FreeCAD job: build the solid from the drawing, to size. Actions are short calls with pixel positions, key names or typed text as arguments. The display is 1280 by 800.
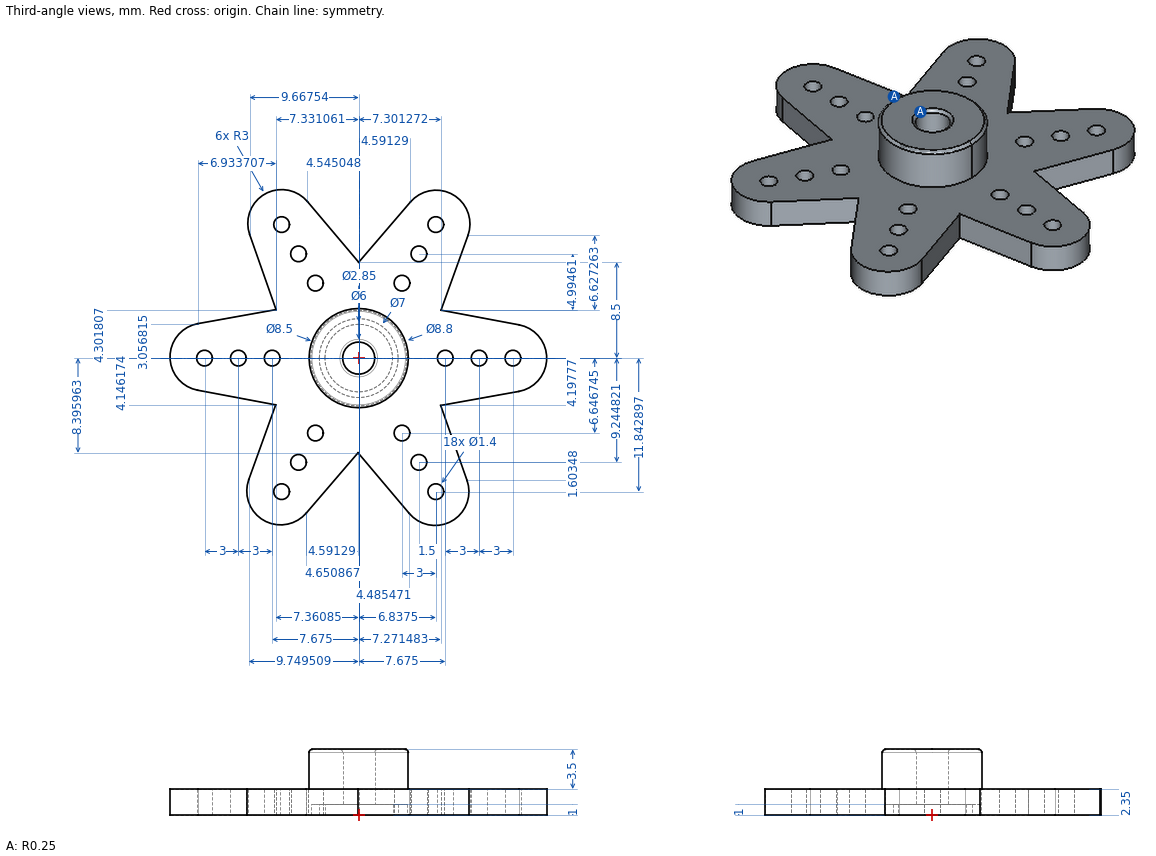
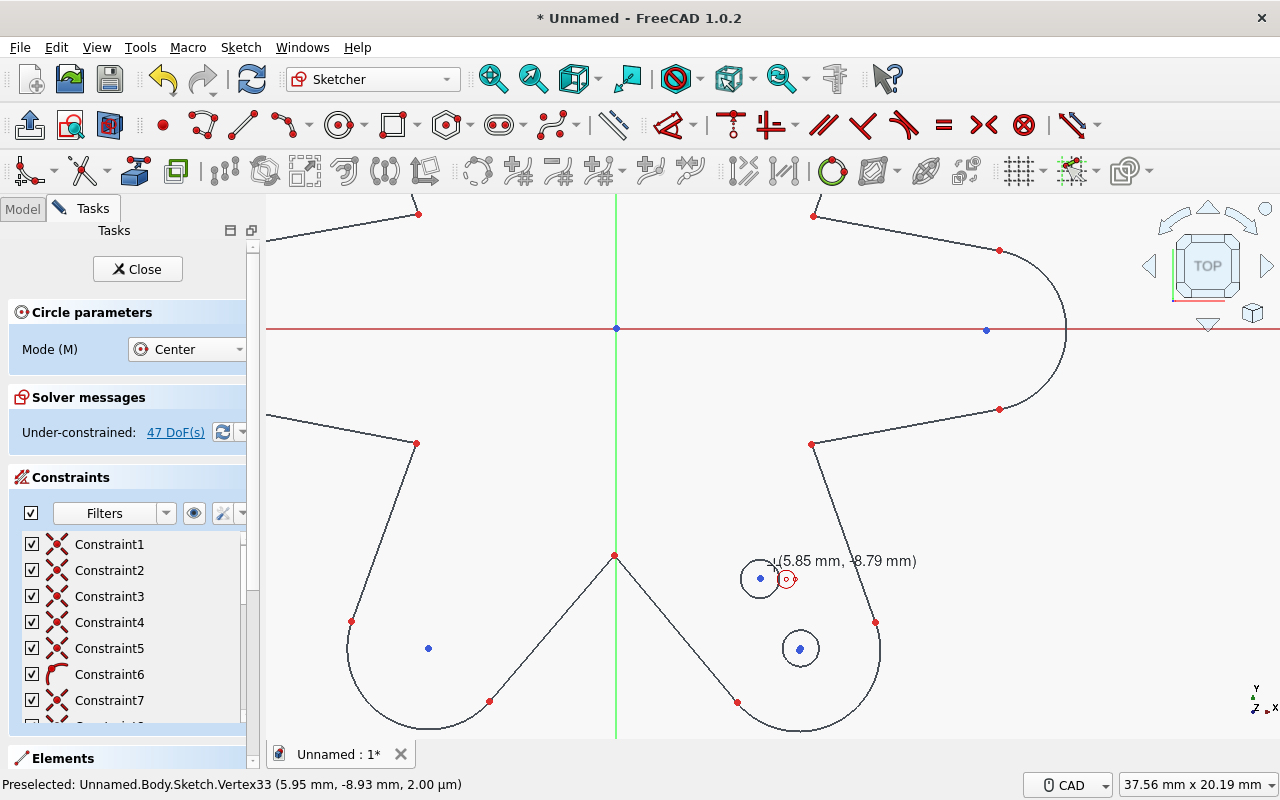
click(720, 508)
click(733, 495)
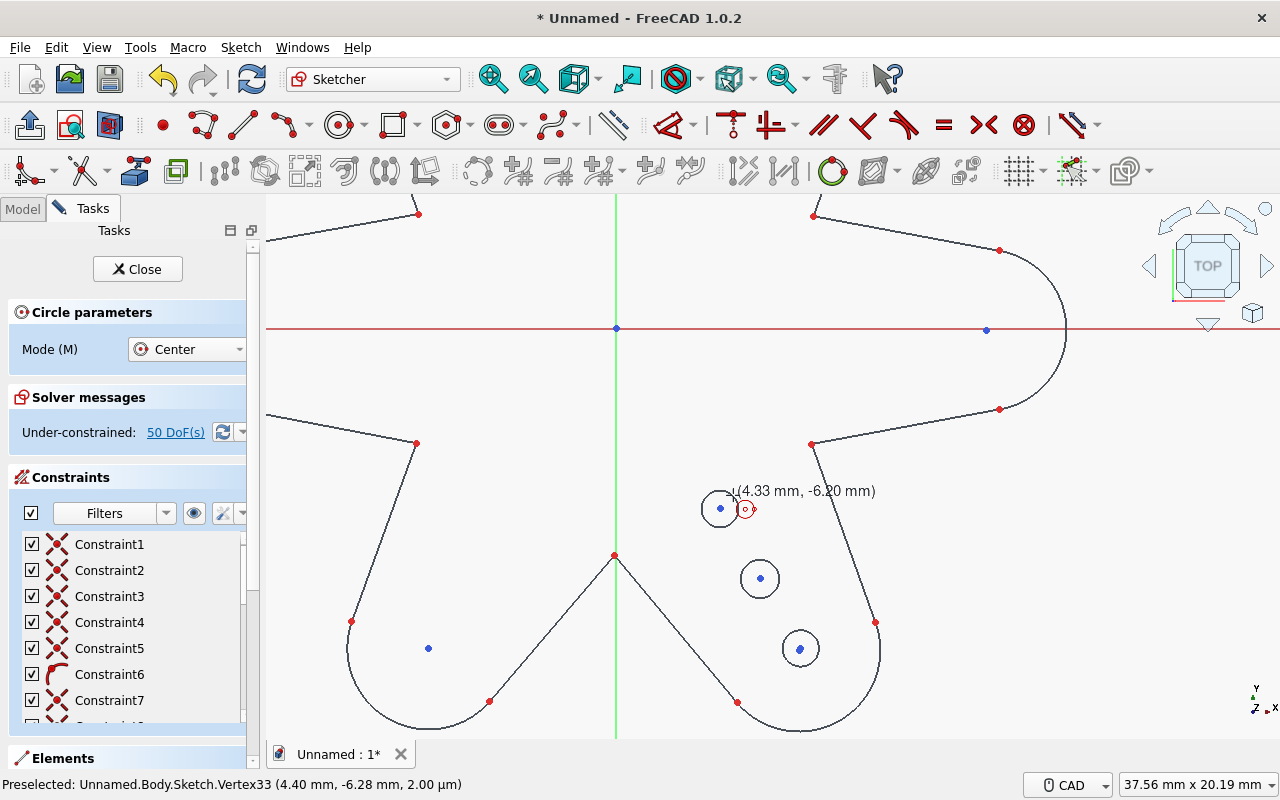
scroll(432, 648, up, 9)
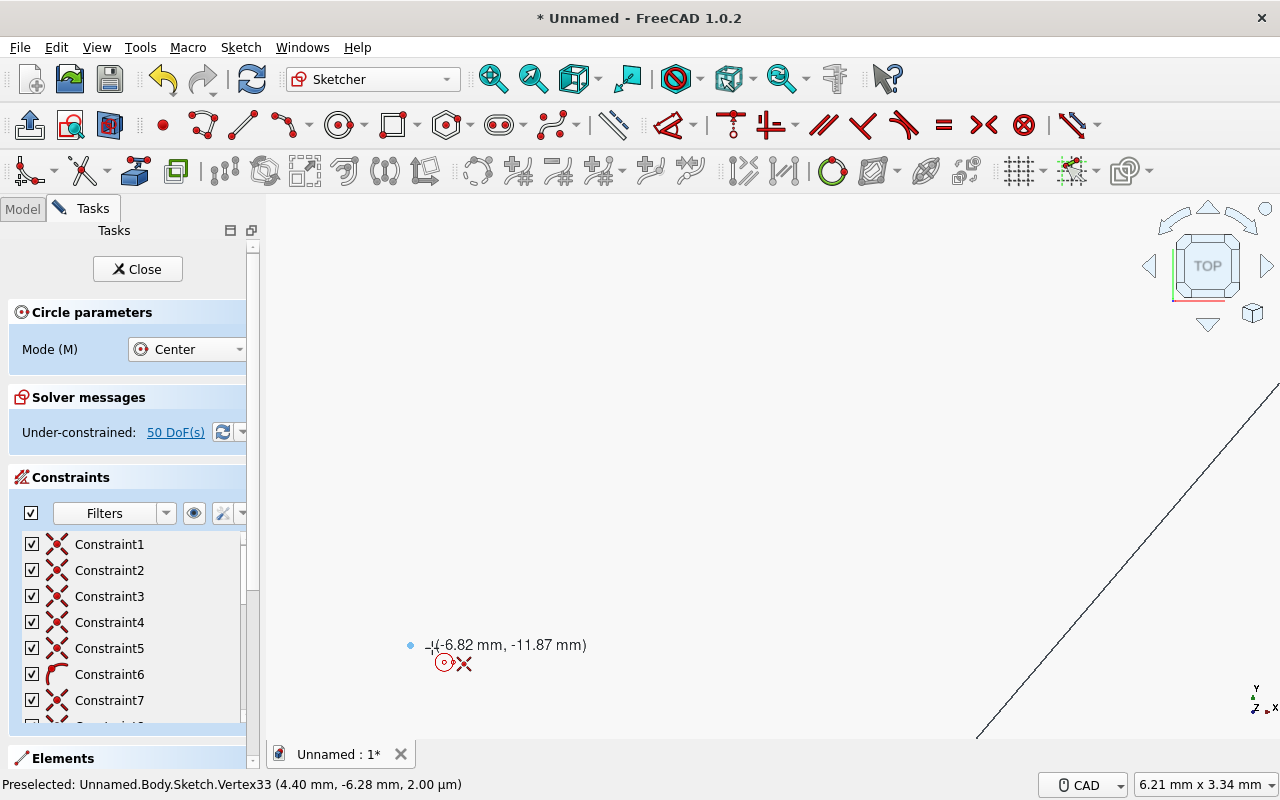
click(428, 646)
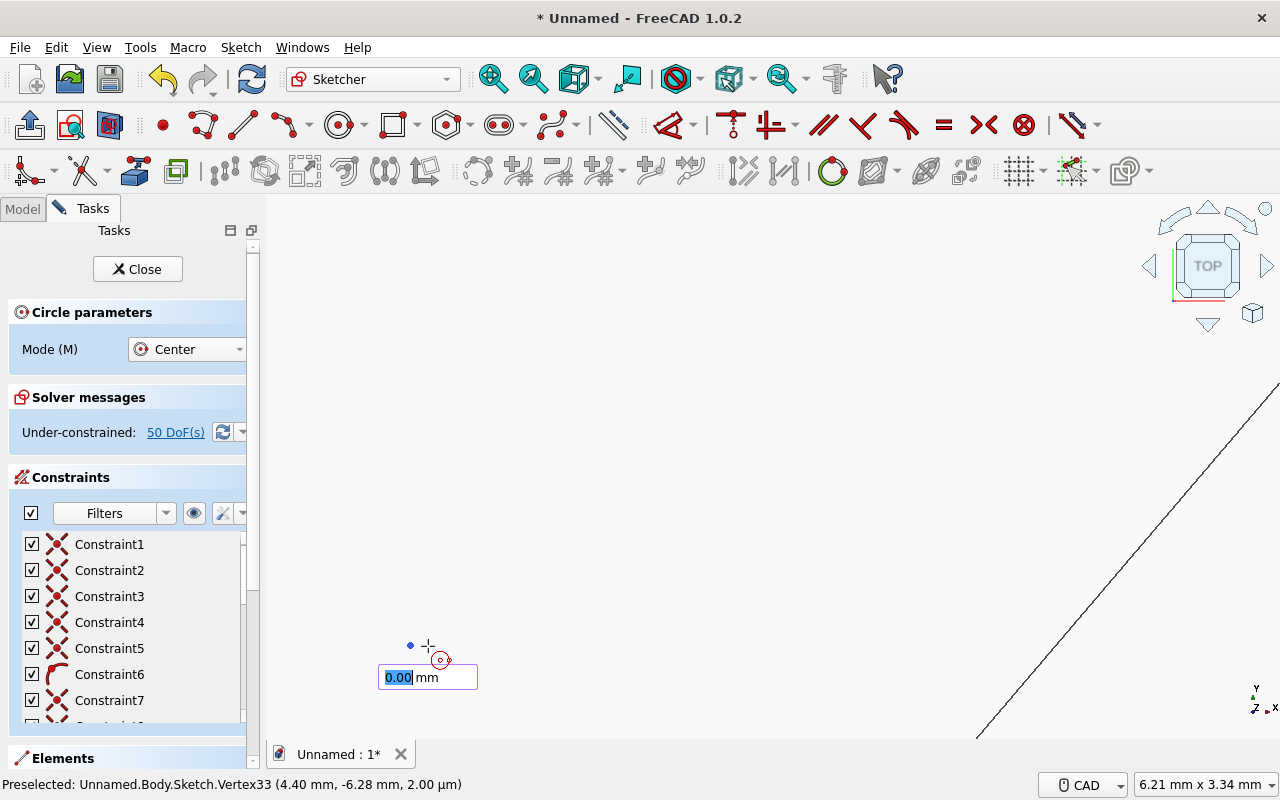
scroll(637, 608, down, 13)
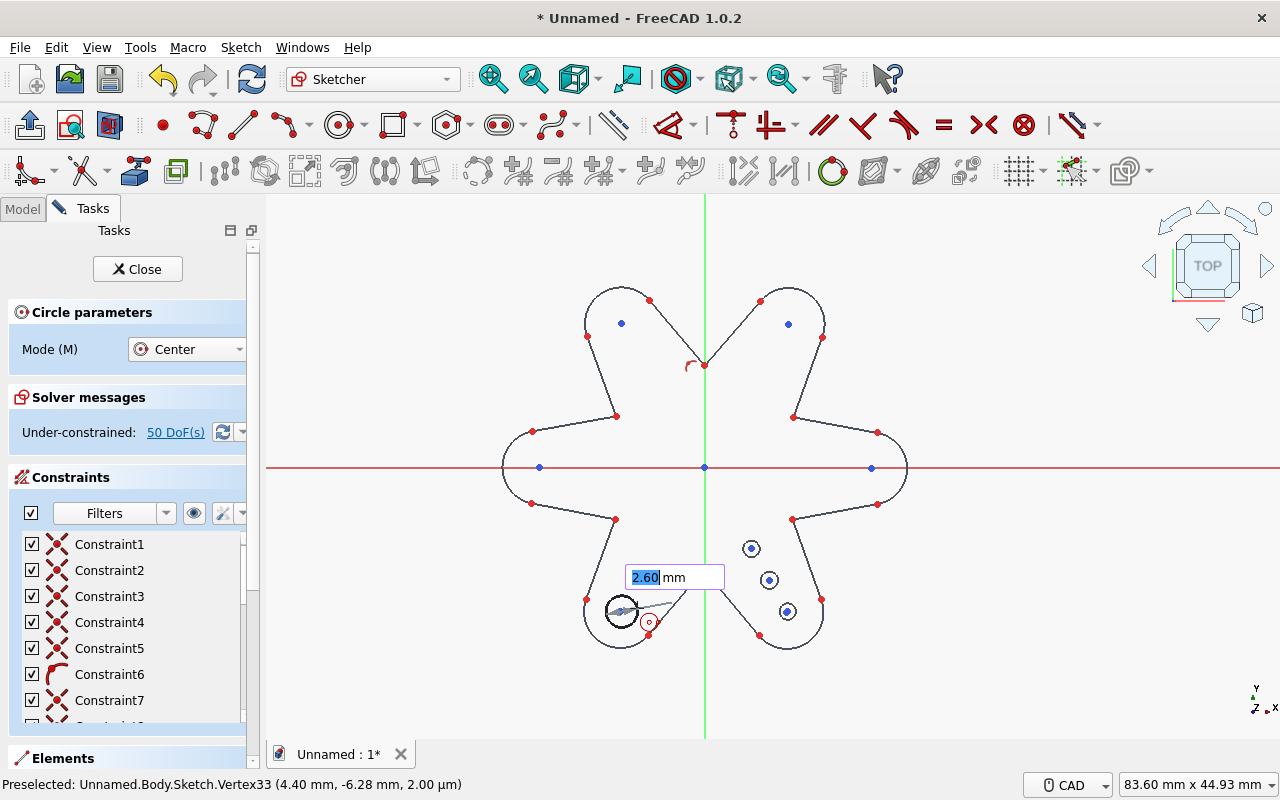
scroll(628, 605, up, 4)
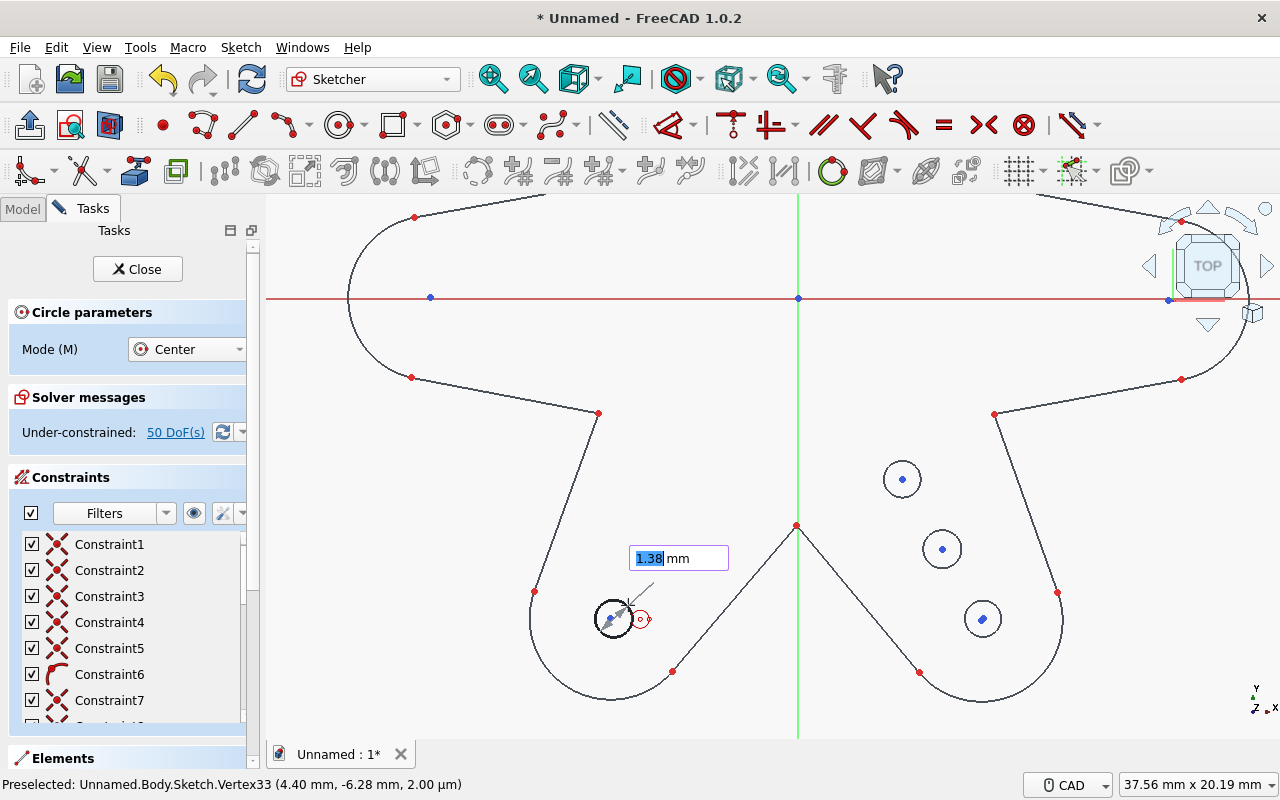
click(627, 605)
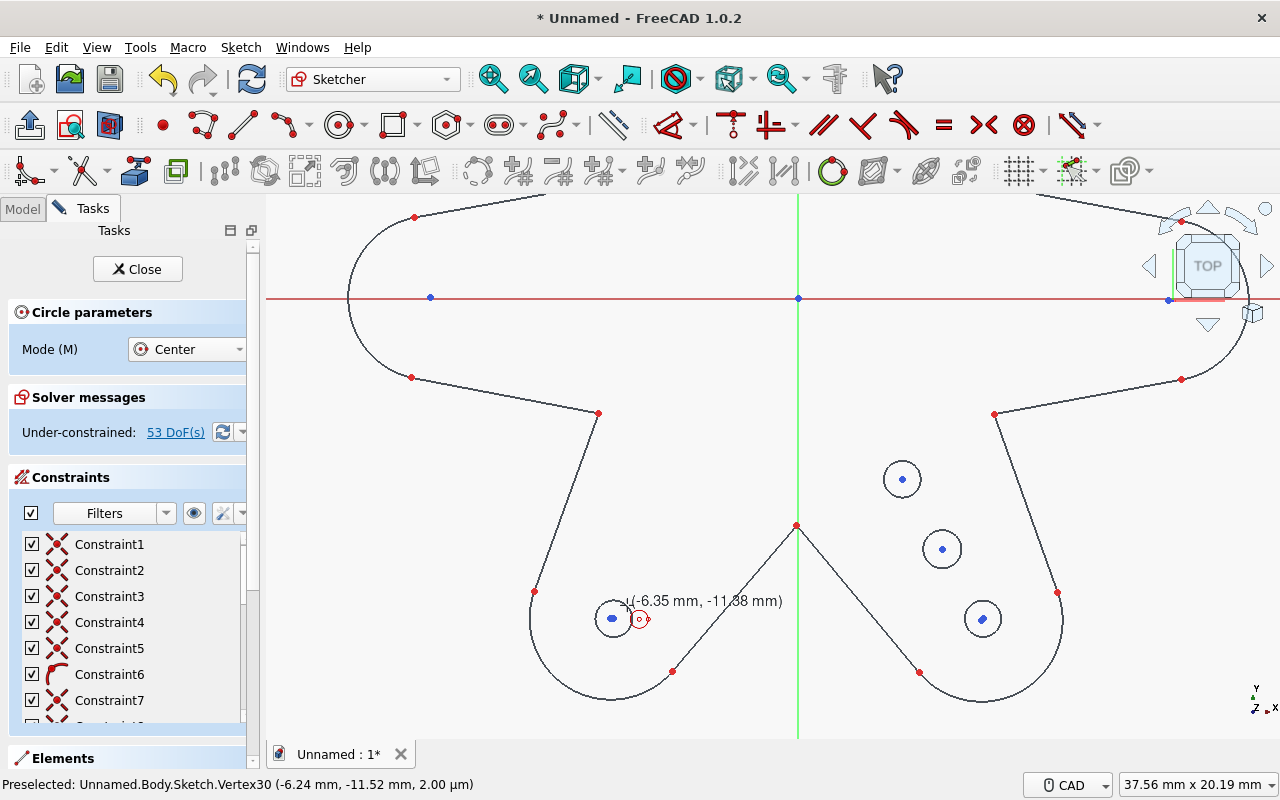
click(654, 548)
click(668, 535)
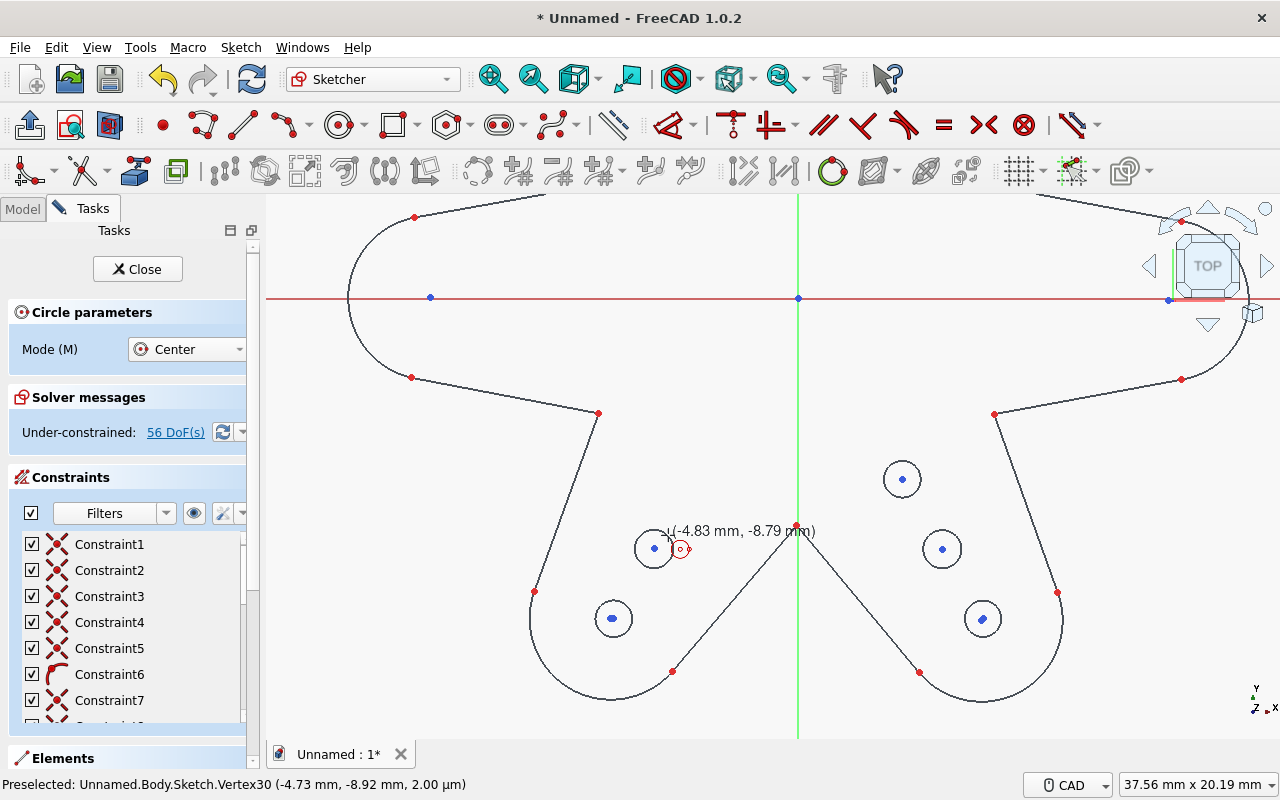
click(695, 478)
click(708, 465)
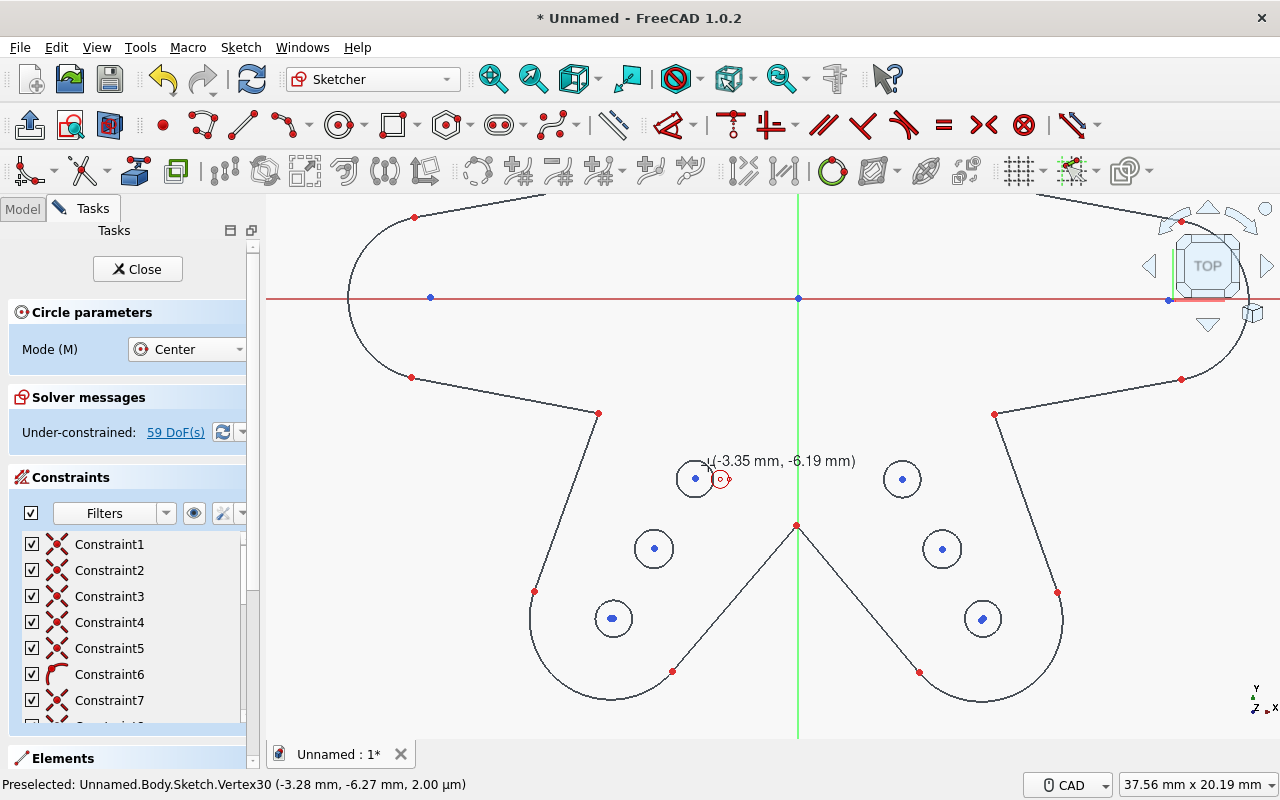
scroll(628, 604, down, 4)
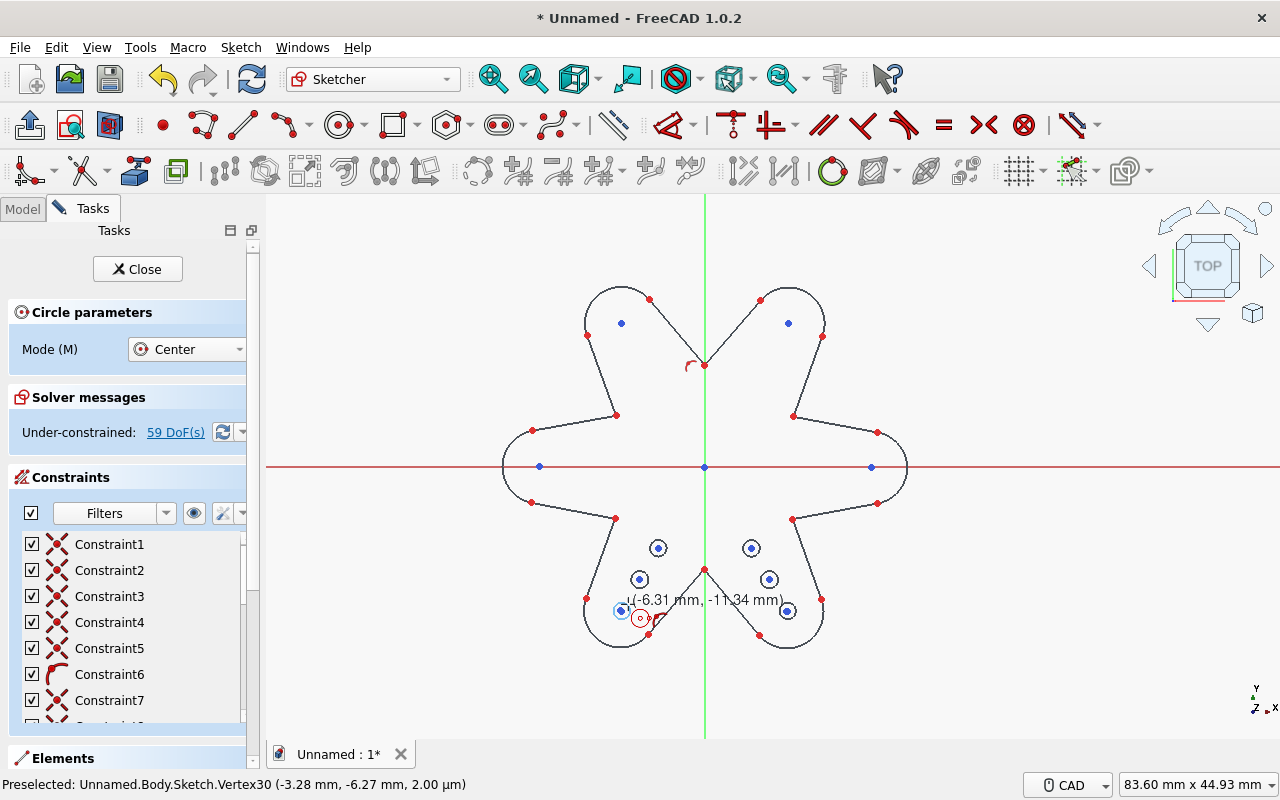
scroll(871, 467, up, 5)